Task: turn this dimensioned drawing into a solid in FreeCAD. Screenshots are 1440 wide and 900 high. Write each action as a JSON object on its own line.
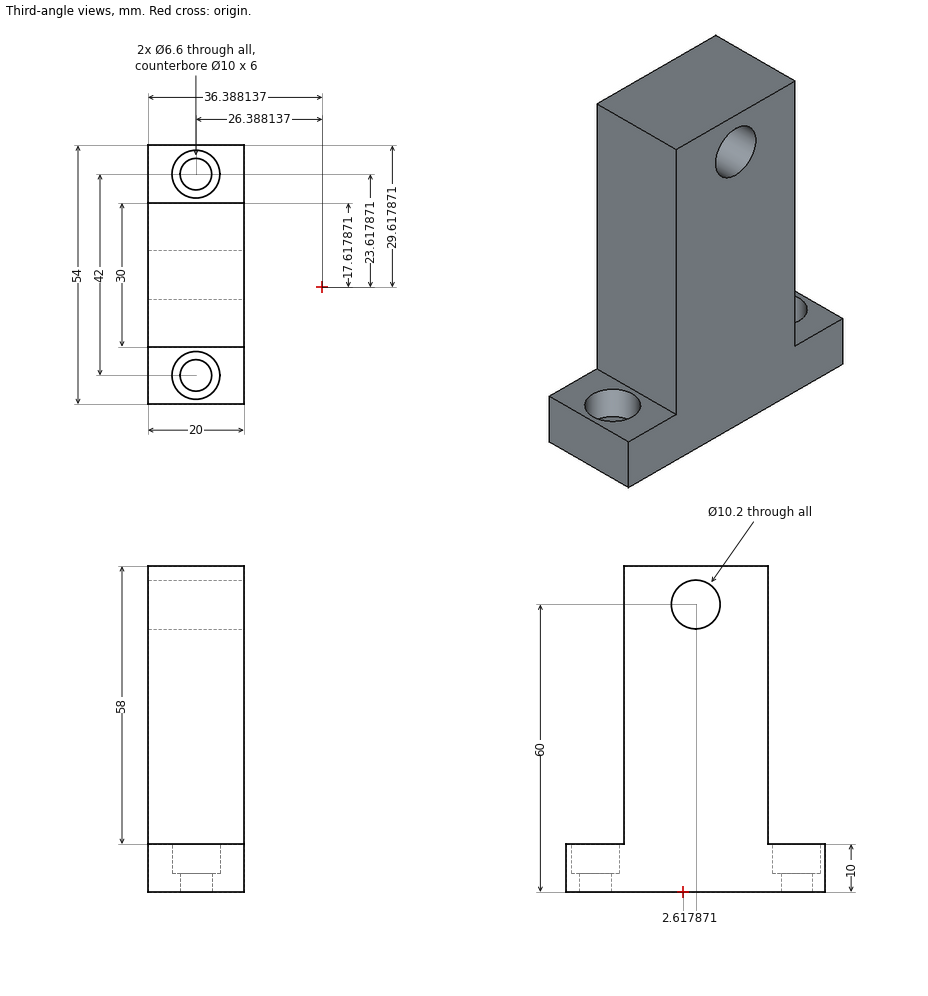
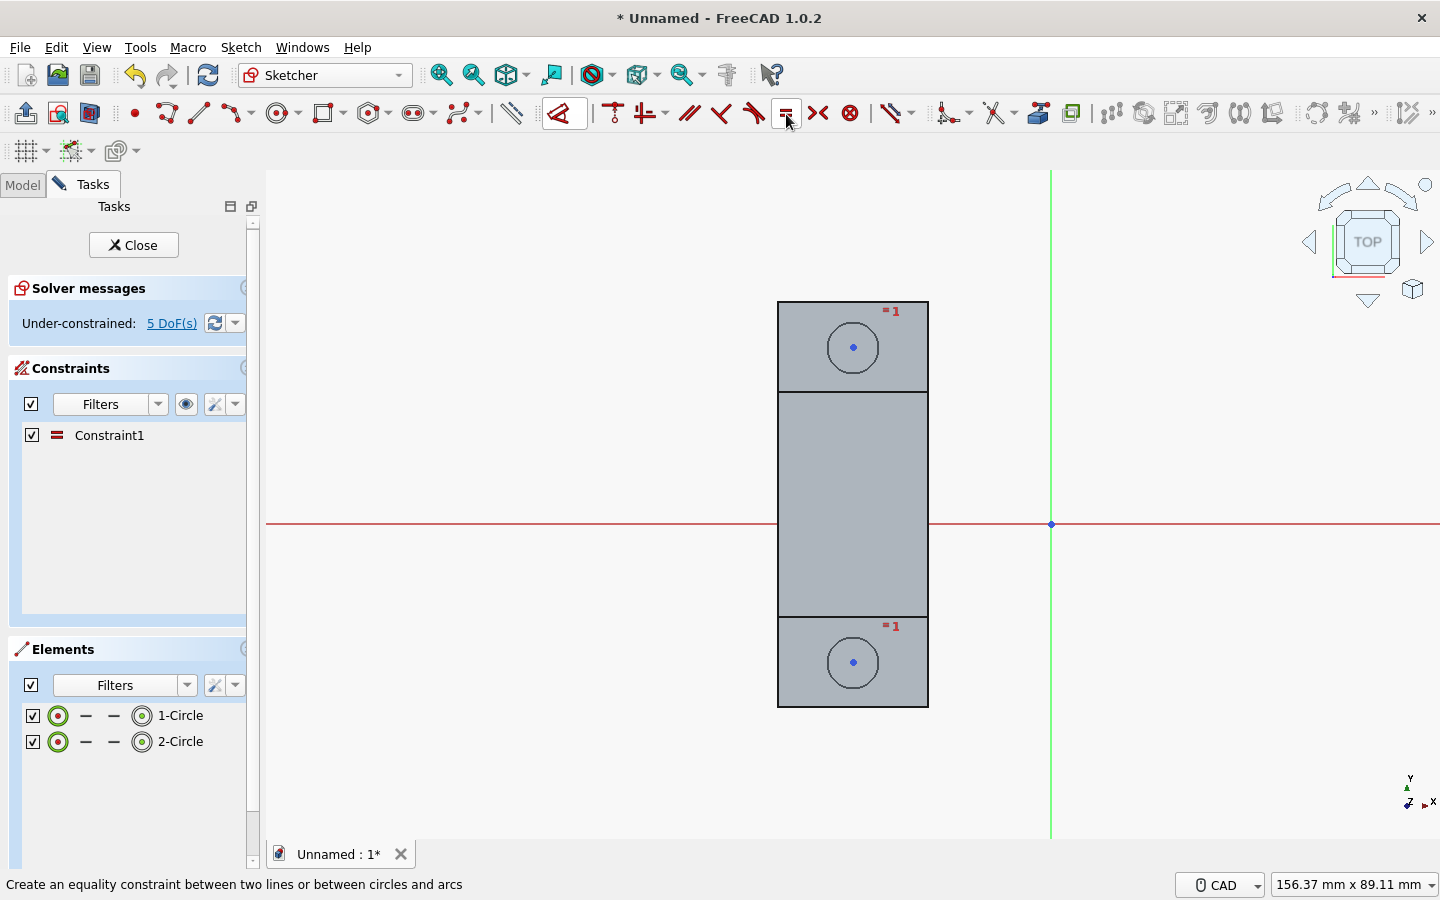
{"action": "left_click", "coordinate": [853, 348]}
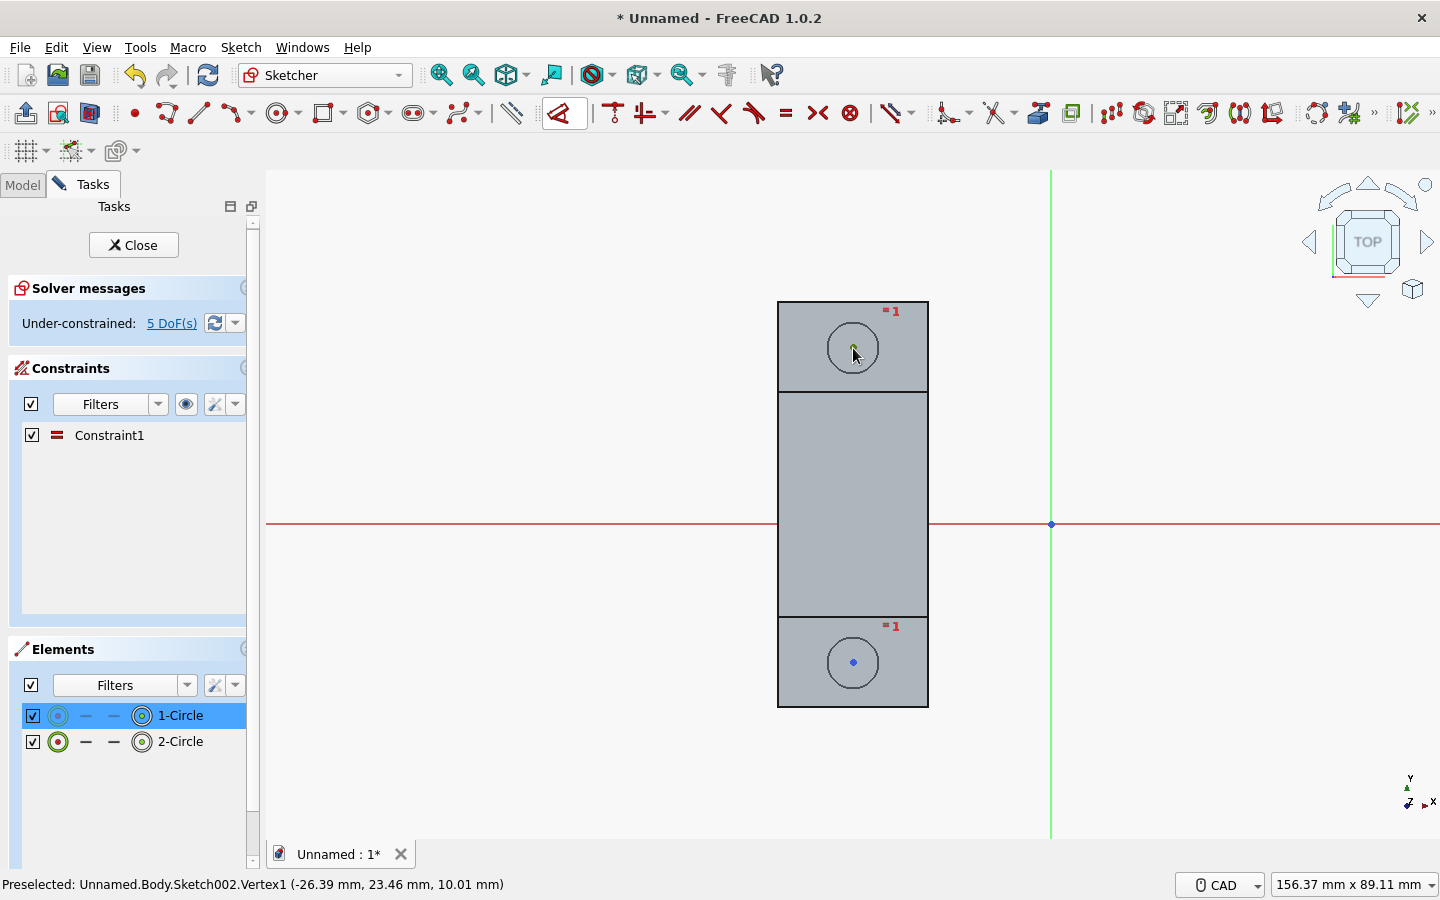
{"action": "left_click", "coordinate": [853, 663]}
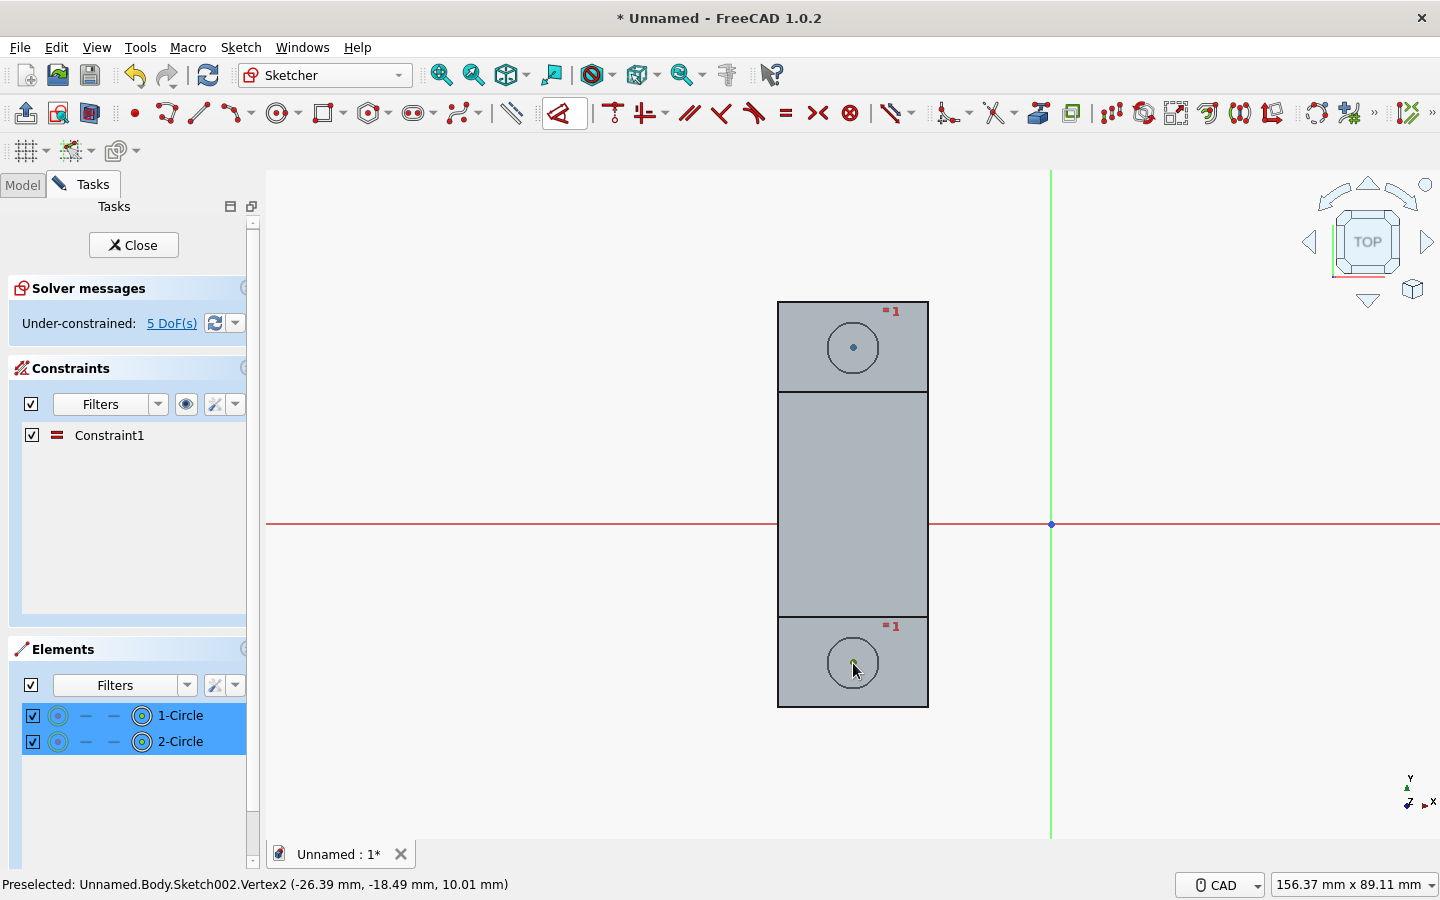
{"action": "key", "text": "v"}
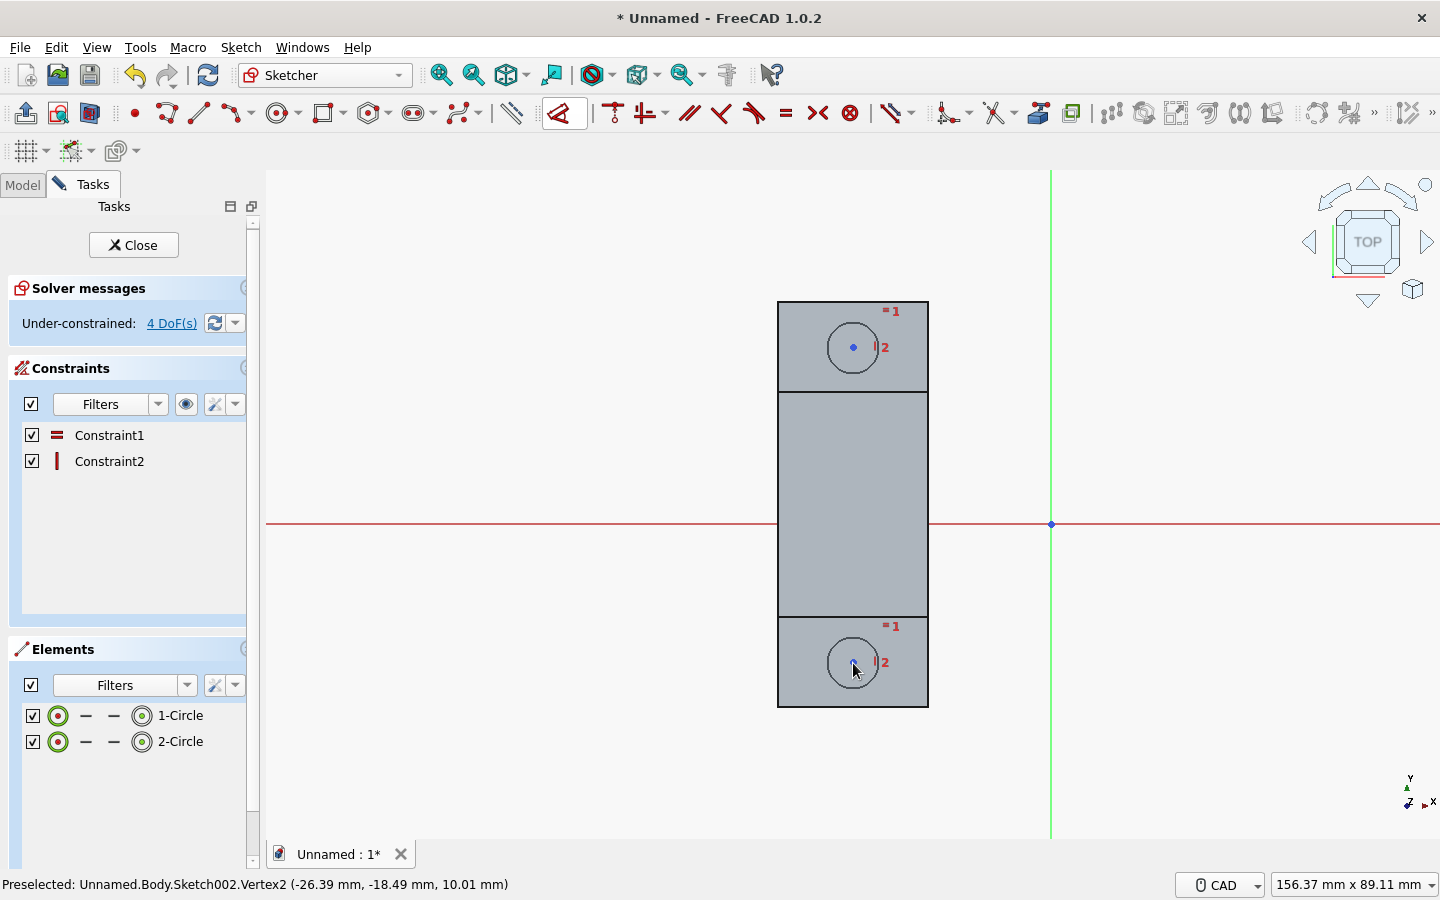
{"action": "left_click", "coordinate": [871, 330]}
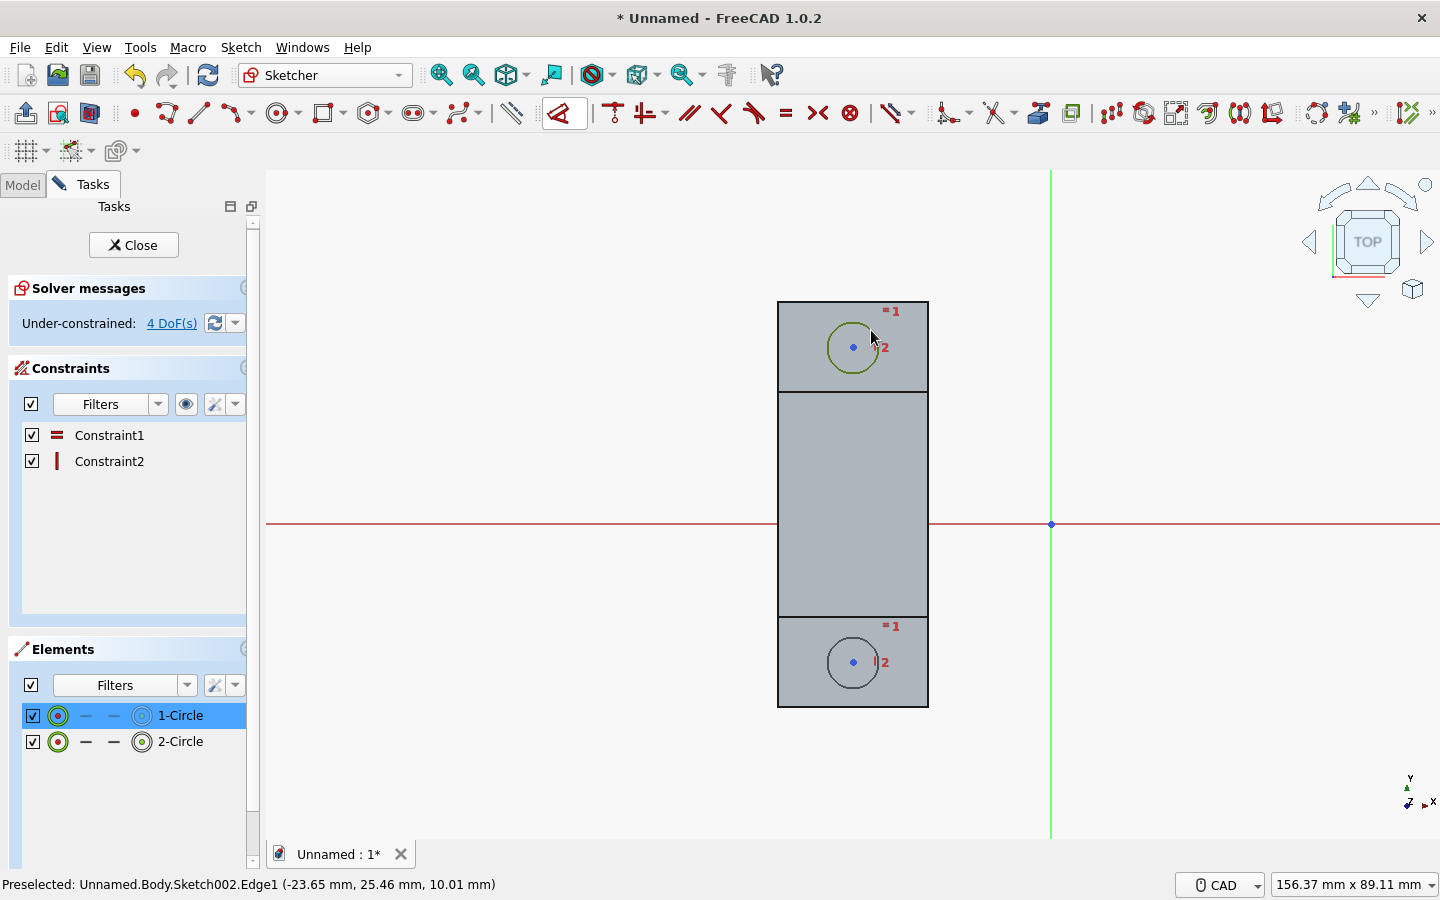
{"action": "key", "text": "k o"}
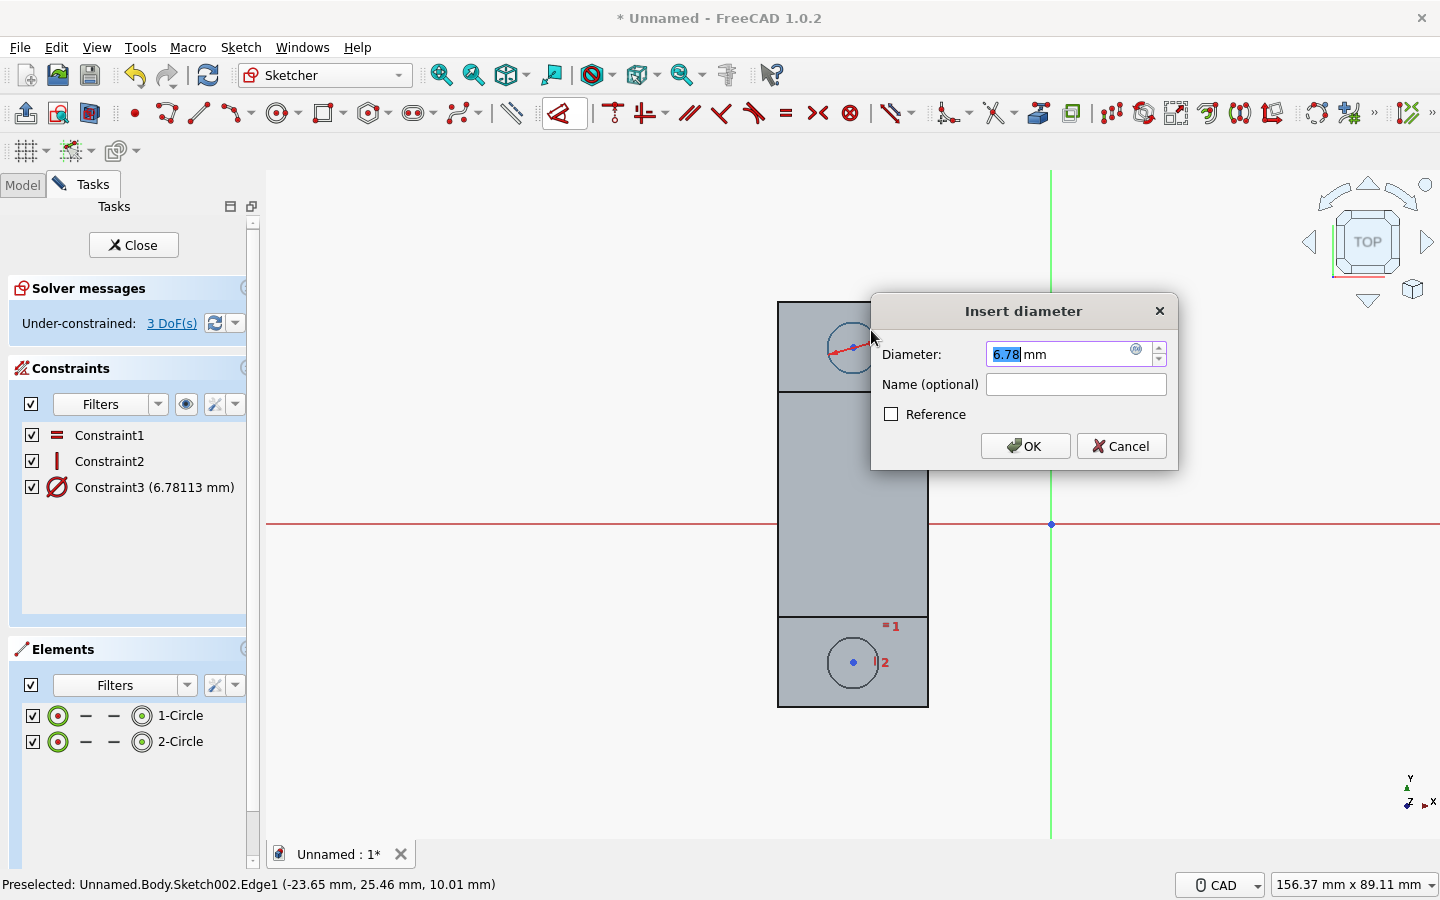
{"action": "type", "text": "6.6"}
{"action": "key", "text": "Return"}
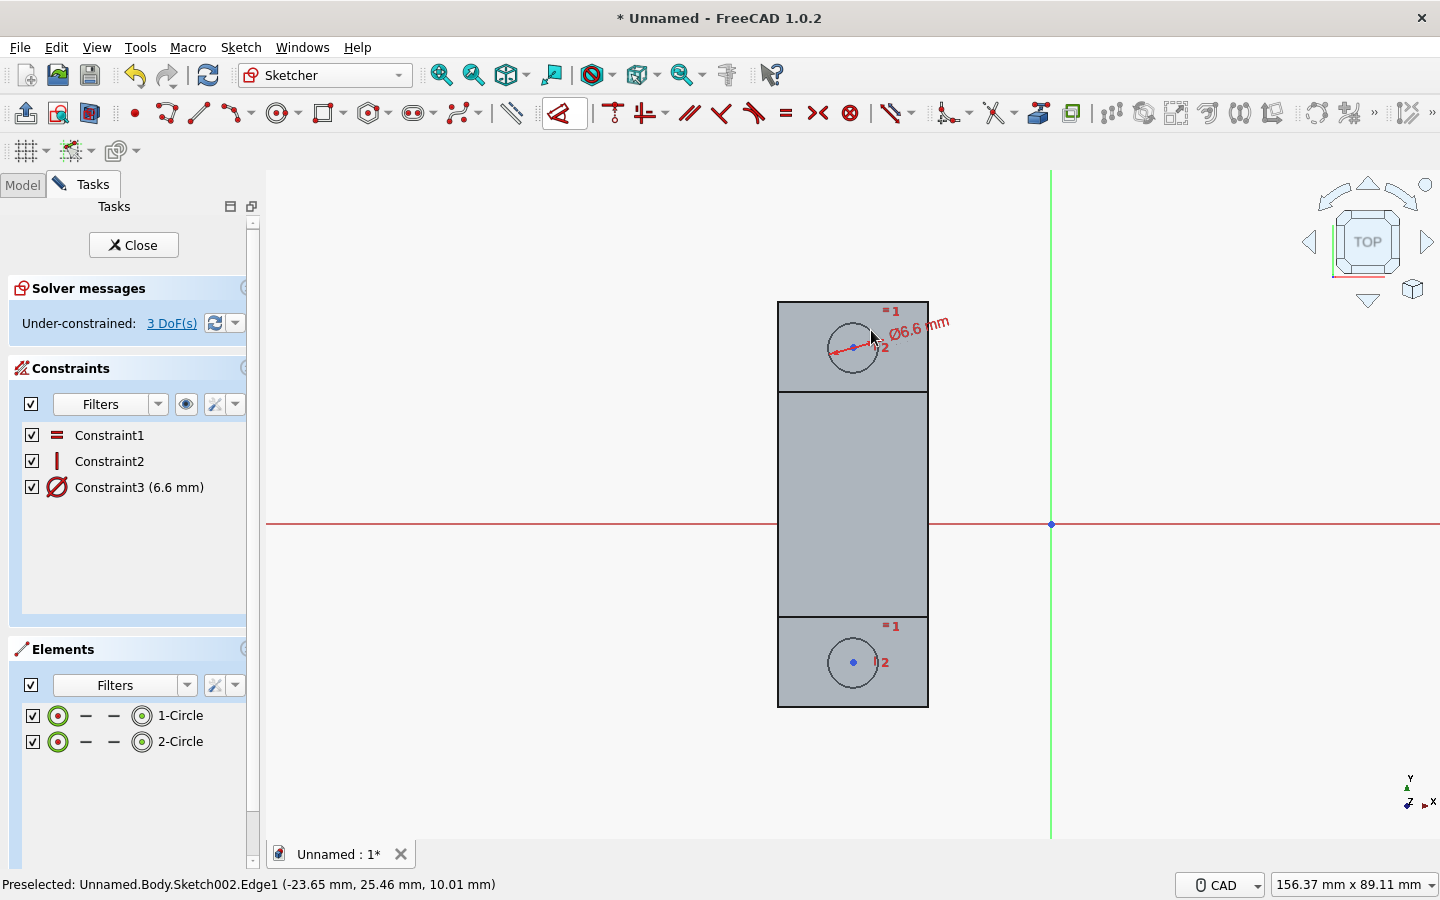
{"action": "left_click", "coordinate": [853, 348]}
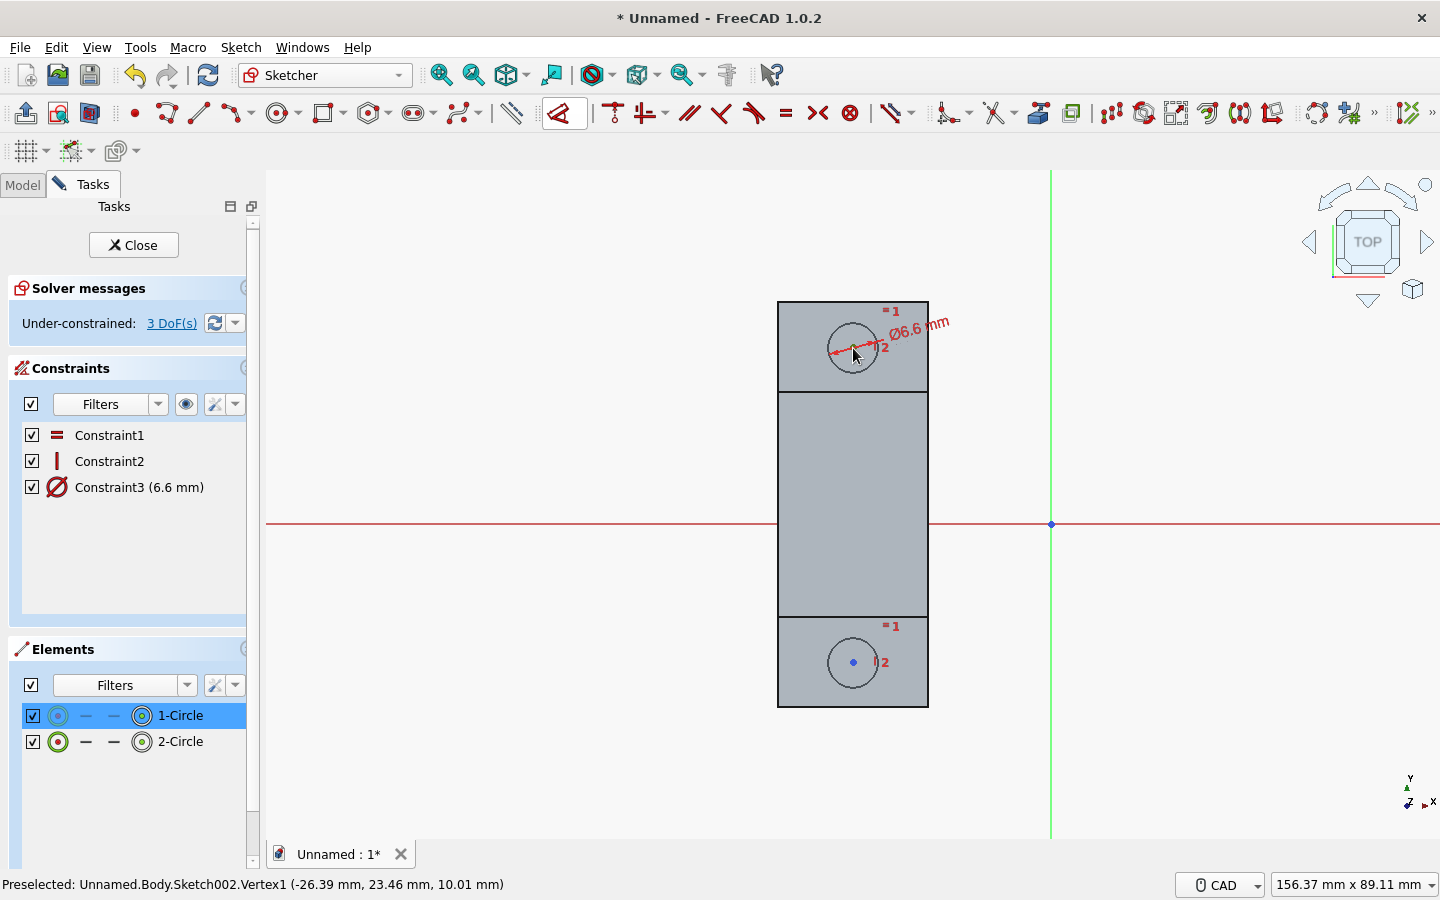
{"action": "left_click", "coordinate": [853, 663]}